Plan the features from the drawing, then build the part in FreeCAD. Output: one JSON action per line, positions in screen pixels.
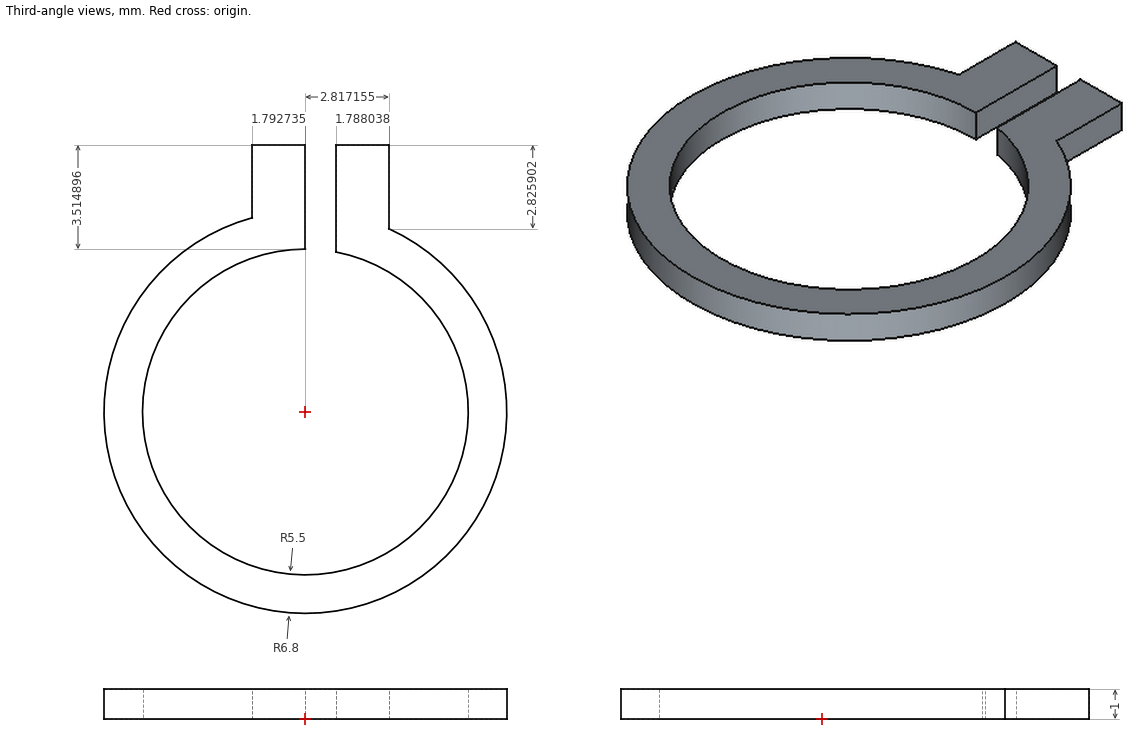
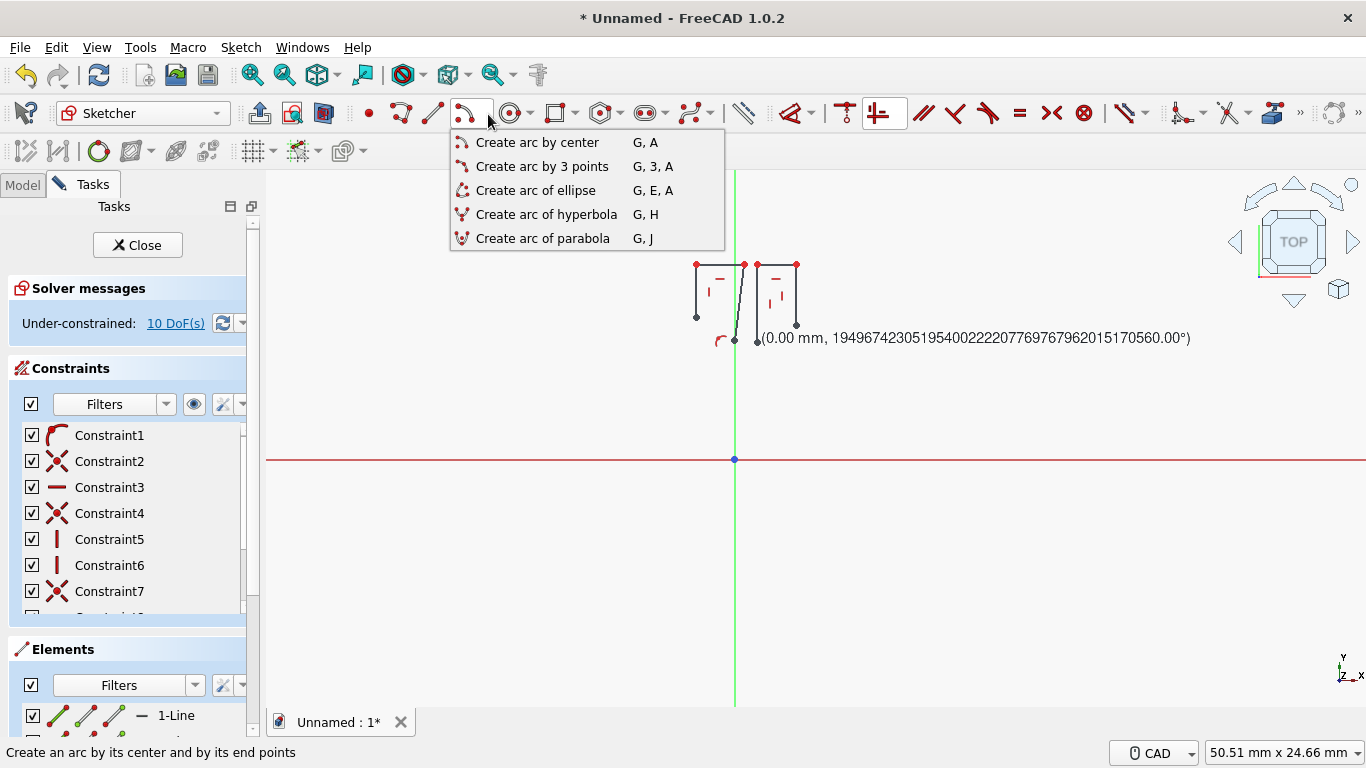
{"action": "left_click", "coordinate": [588, 166]}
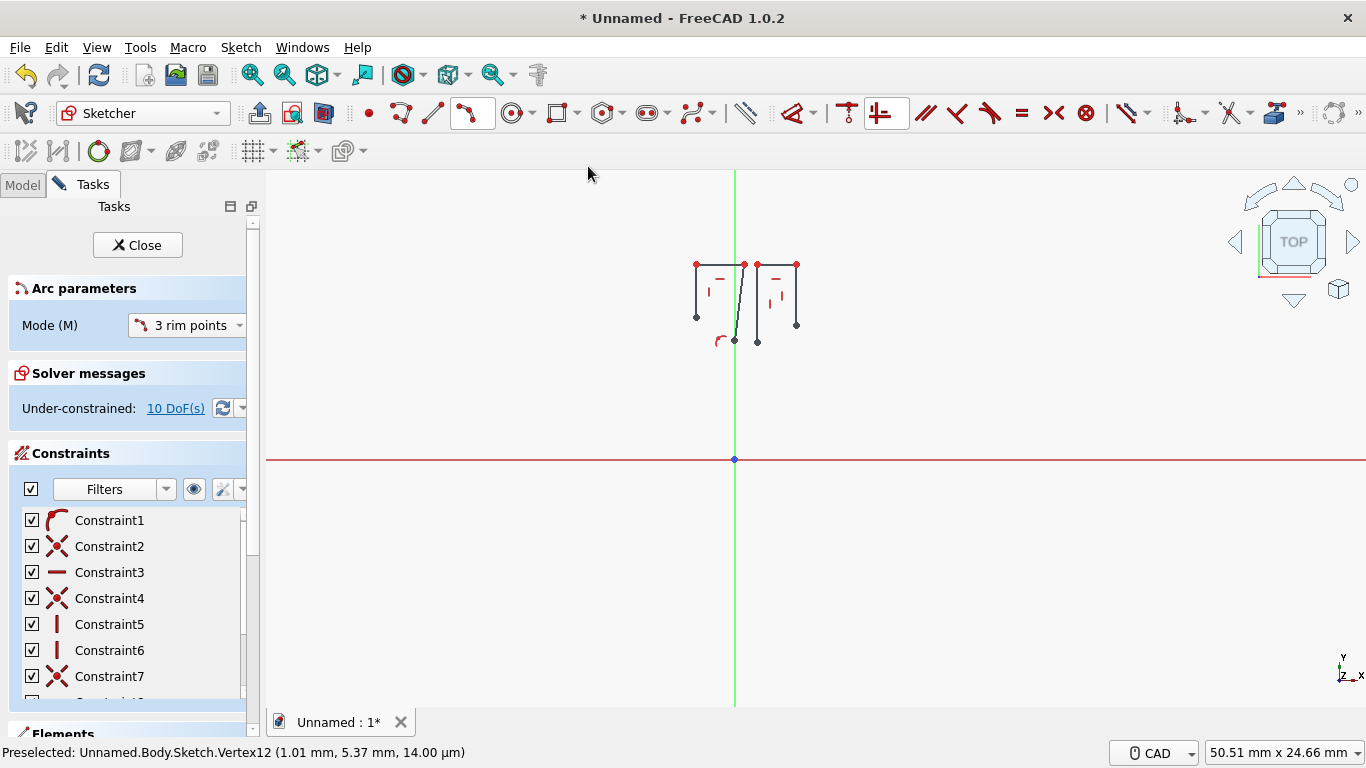
{"action": "left_click", "coordinate": [696, 318]}
{"action": "left_click", "coordinate": [796, 326]}
{"action": "left_click", "coordinate": [647, 579]}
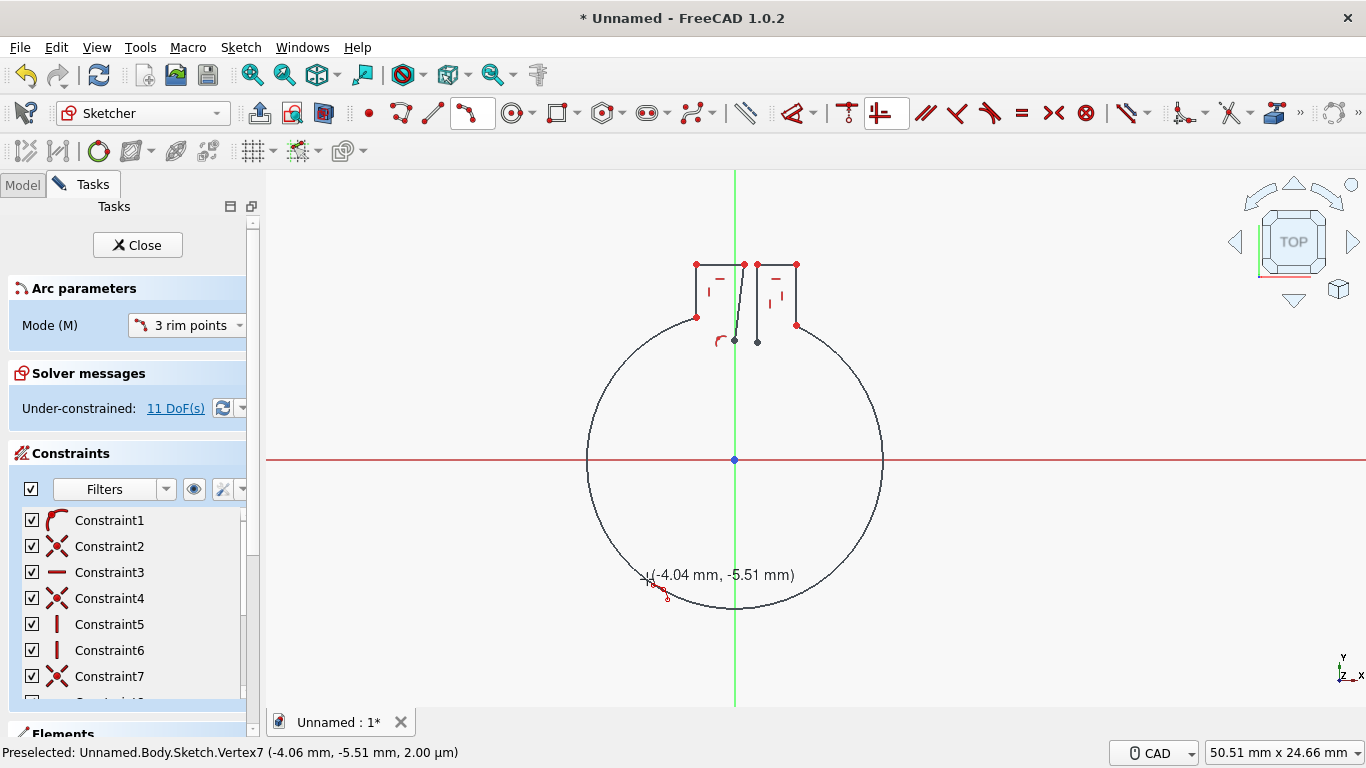
{"action": "left_click", "coordinate": [757, 343]}
{"action": "left_click", "coordinate": [735, 341]}
{"action": "left_click", "coordinate": [657, 551]}
{"action": "key", "text": "Escape"}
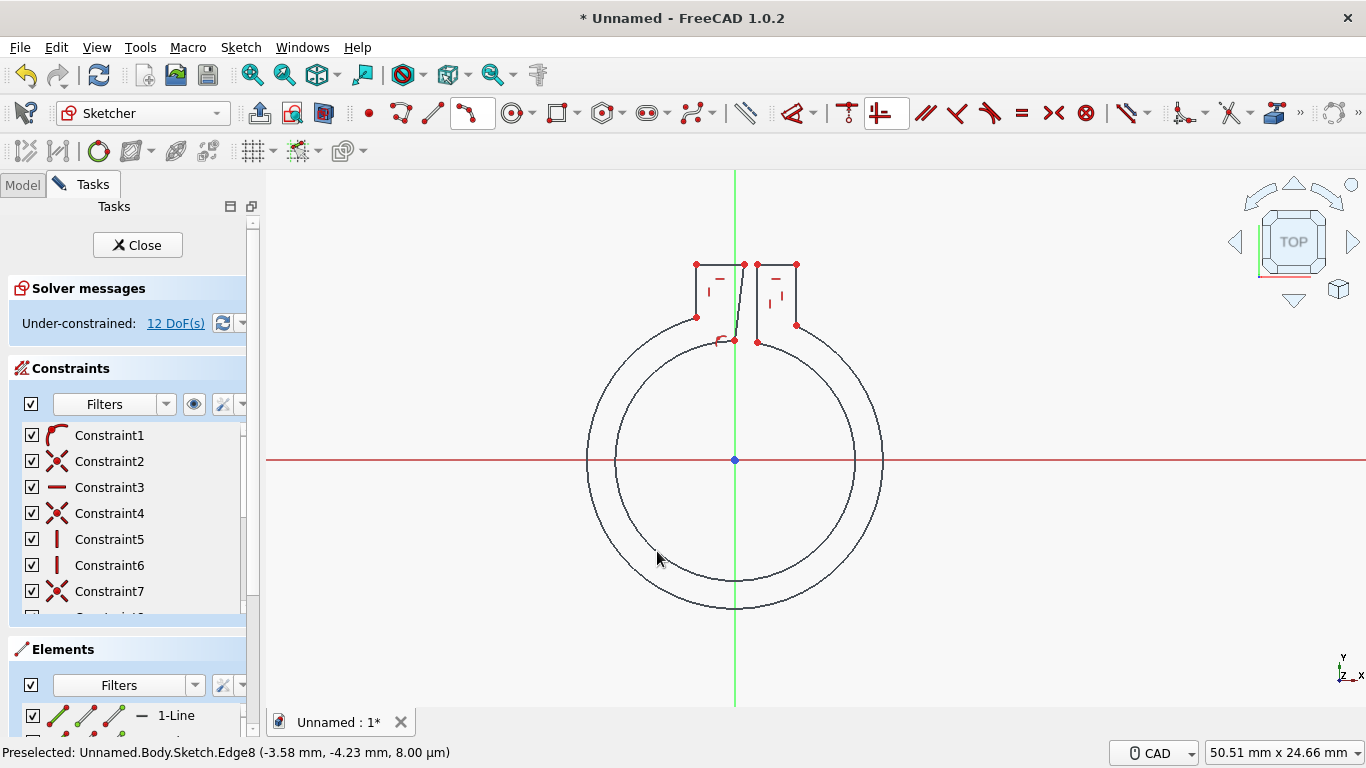
{"action": "left_click", "coordinate": [738, 318]}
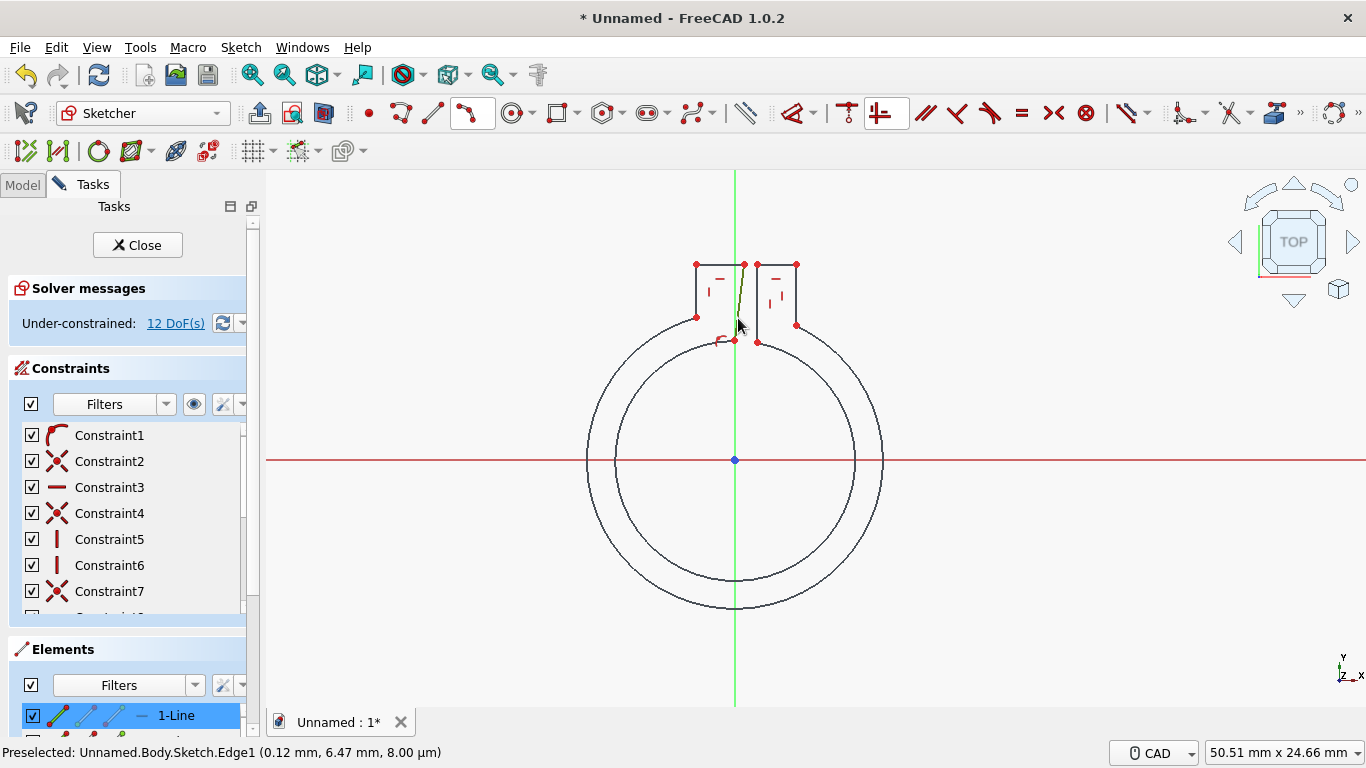
{"action": "left_click", "coordinate": [904, 114]}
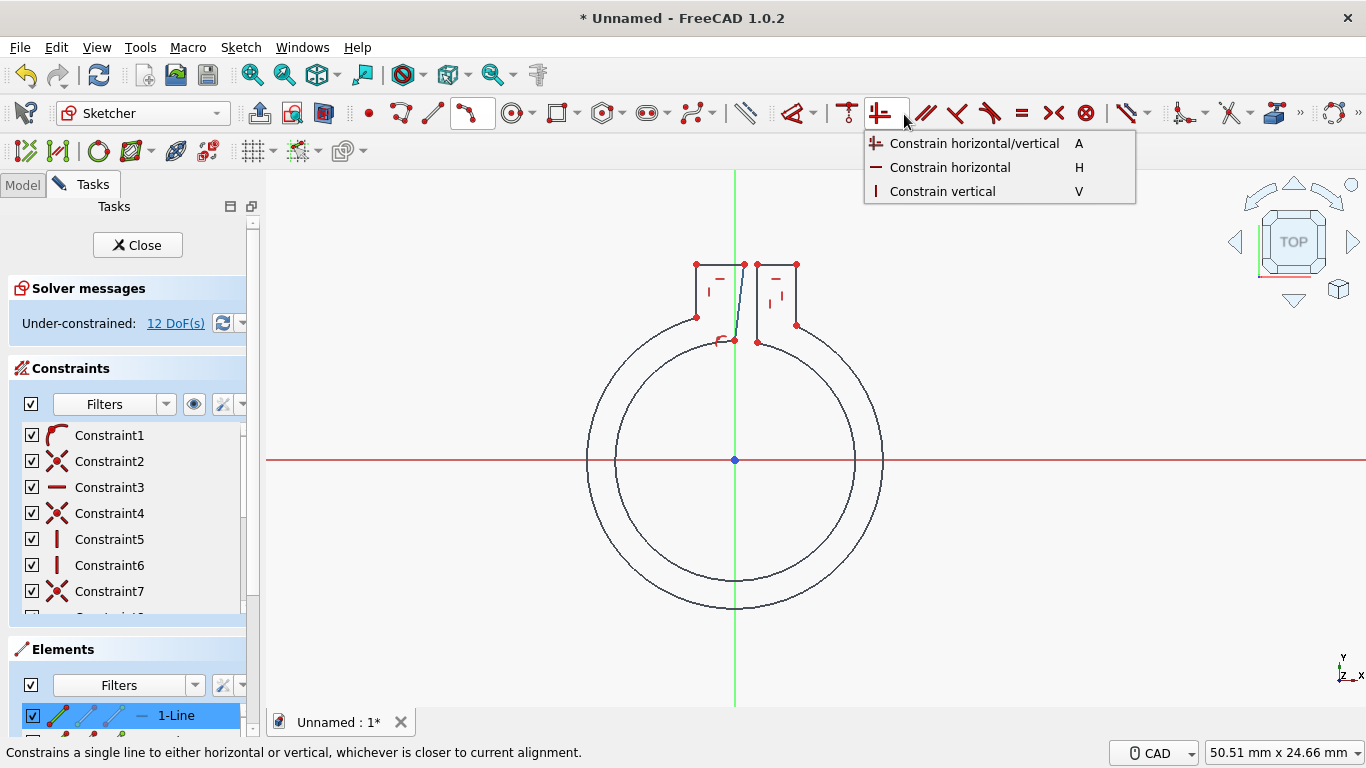
{"action": "left_click", "coordinate": [1000, 191]}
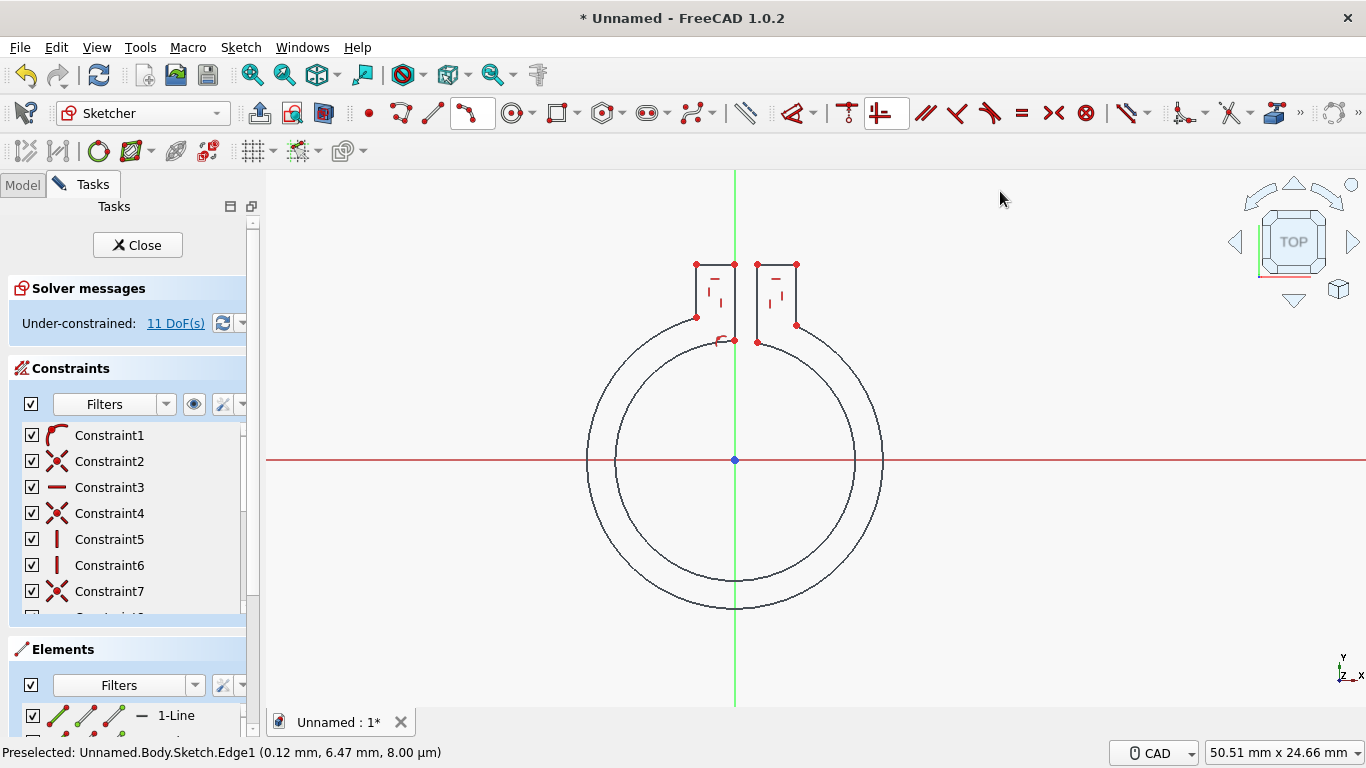
{"action": "left_click", "coordinate": [597, 515]}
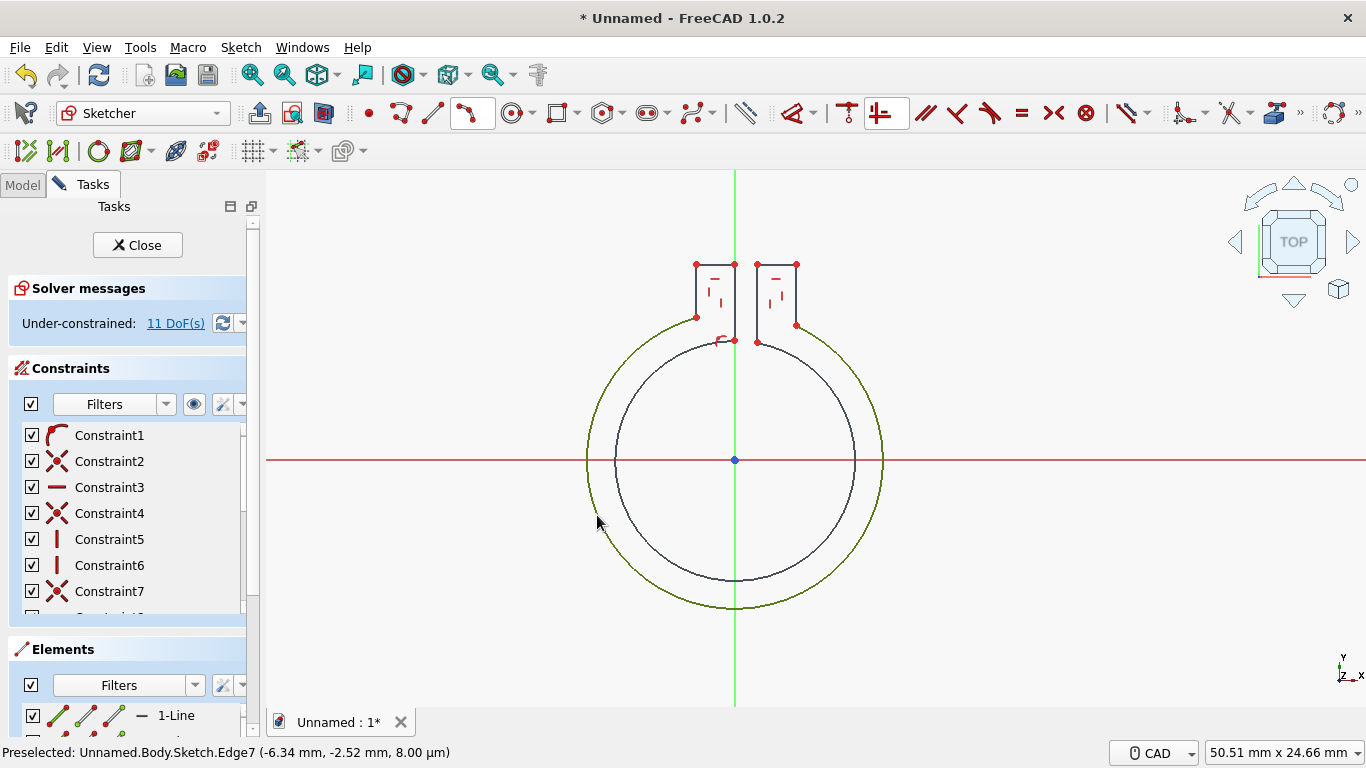
{"action": "left_click", "coordinate": [619, 492]}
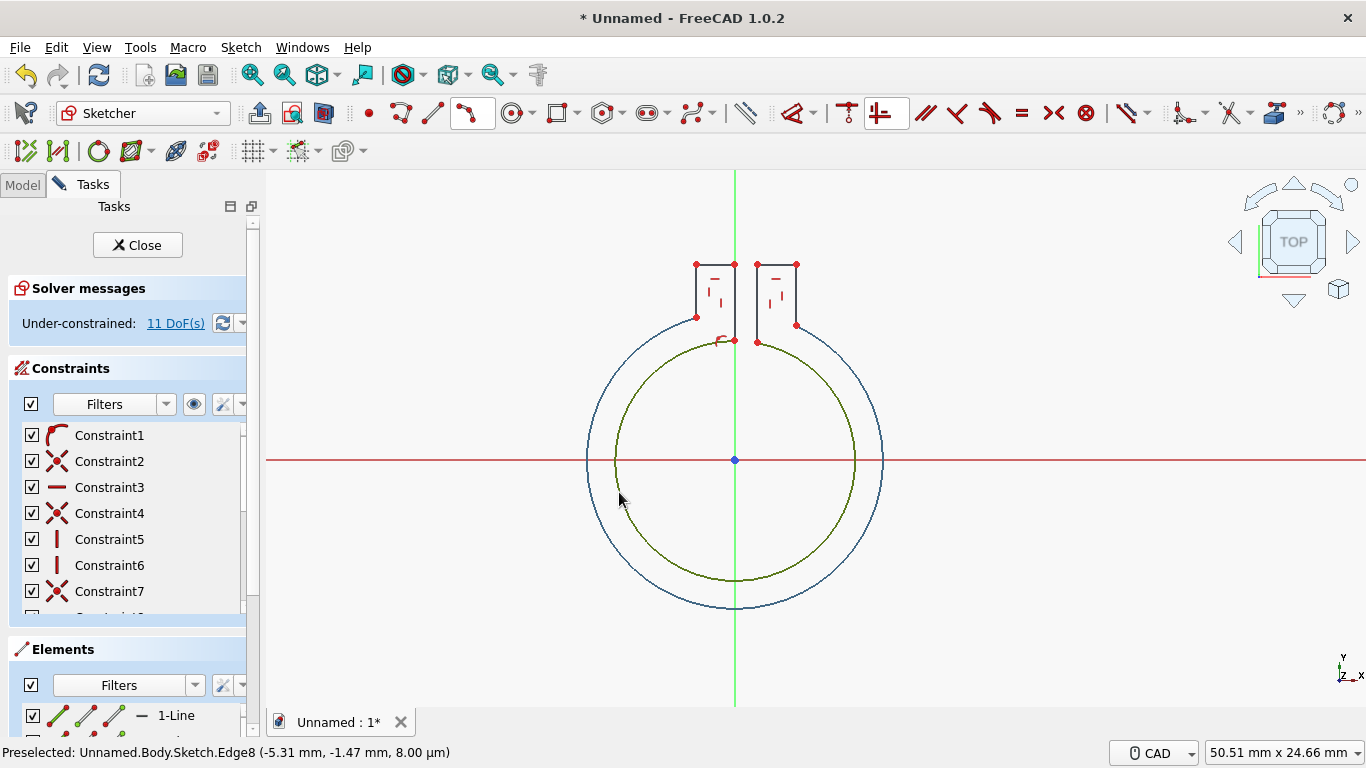
{"action": "left_click", "coordinate": [848, 114]}